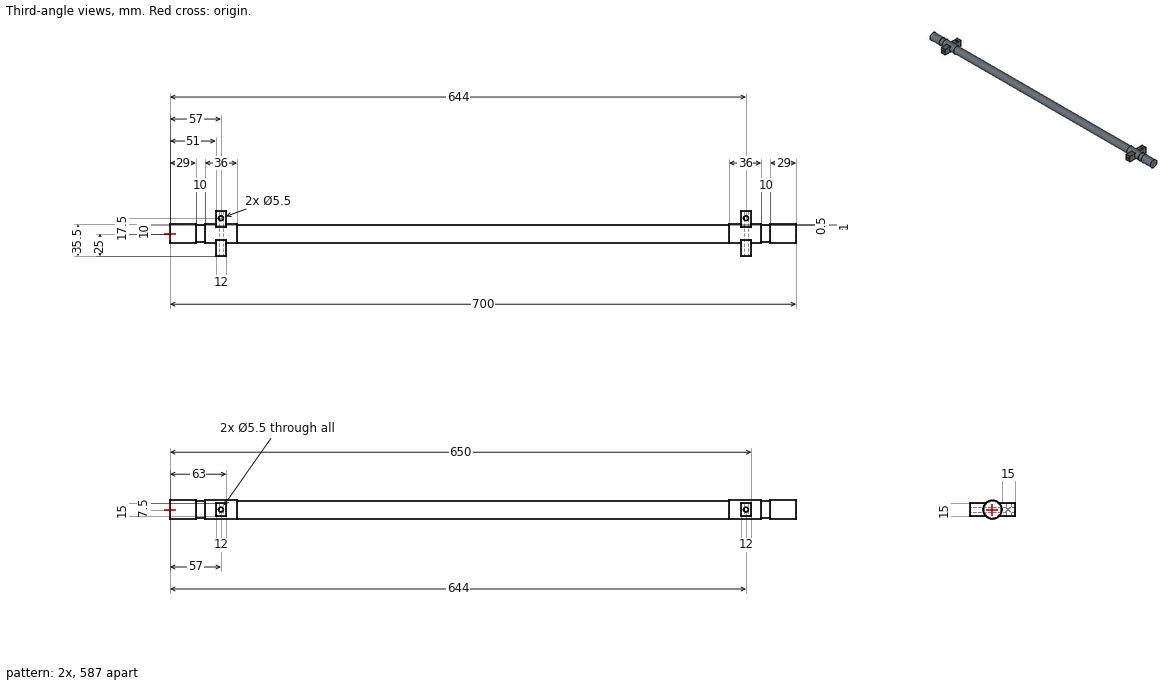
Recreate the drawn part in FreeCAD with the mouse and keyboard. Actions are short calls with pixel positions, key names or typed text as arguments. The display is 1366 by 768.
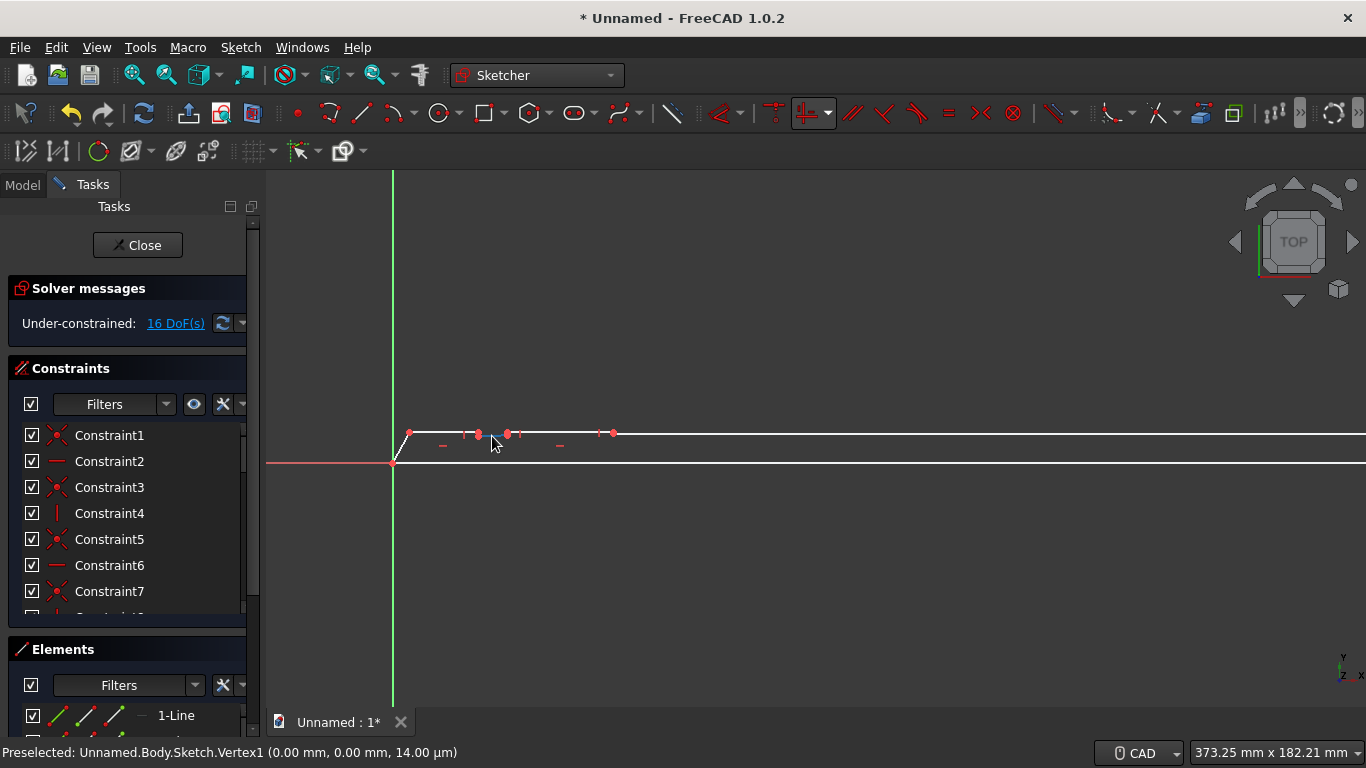
click(493, 436)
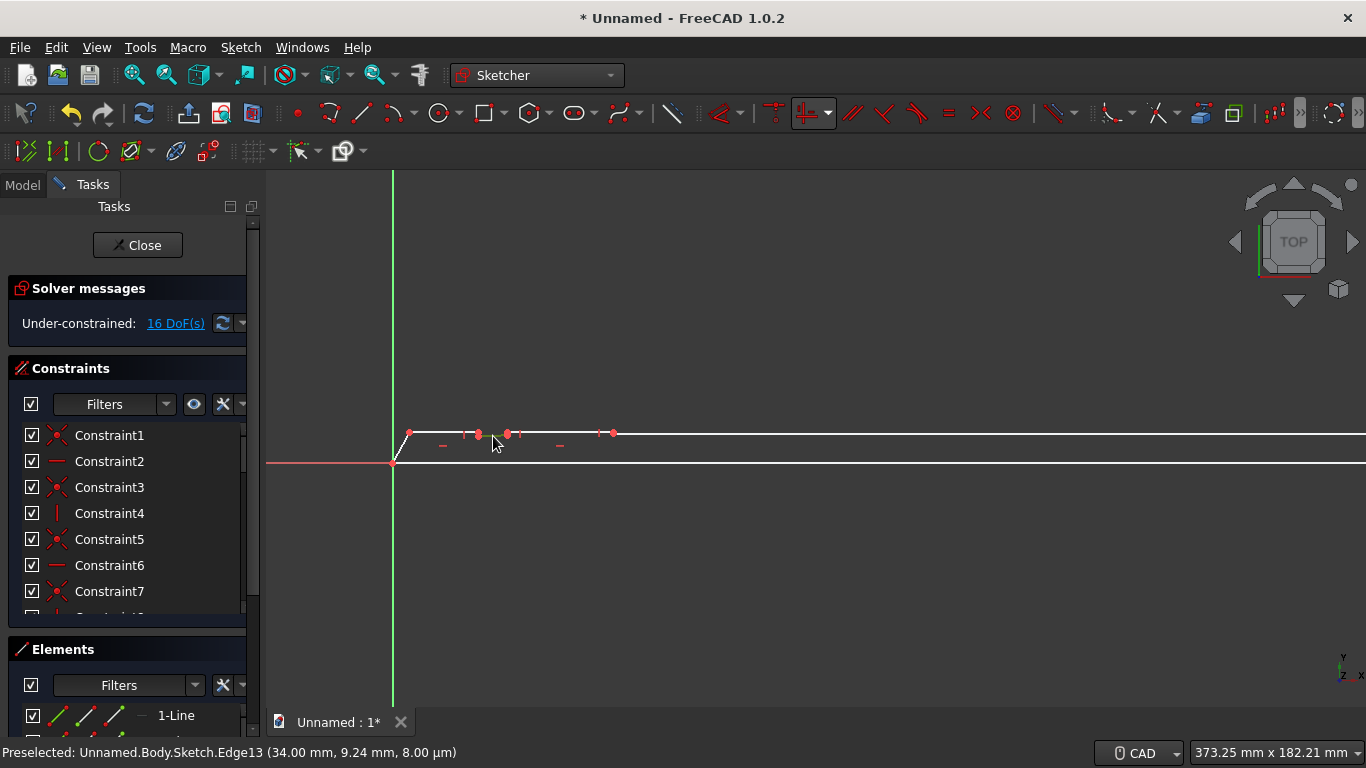
click(830, 114)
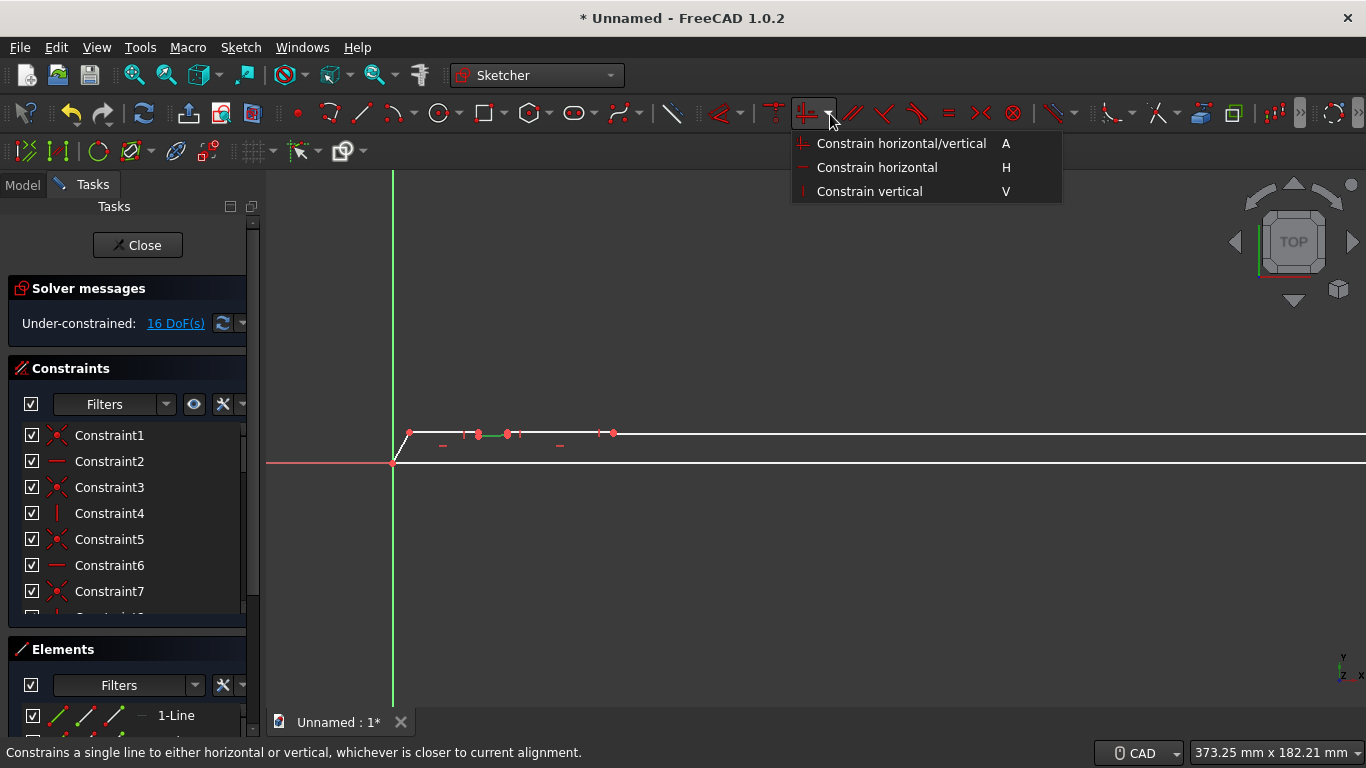
click(927, 167)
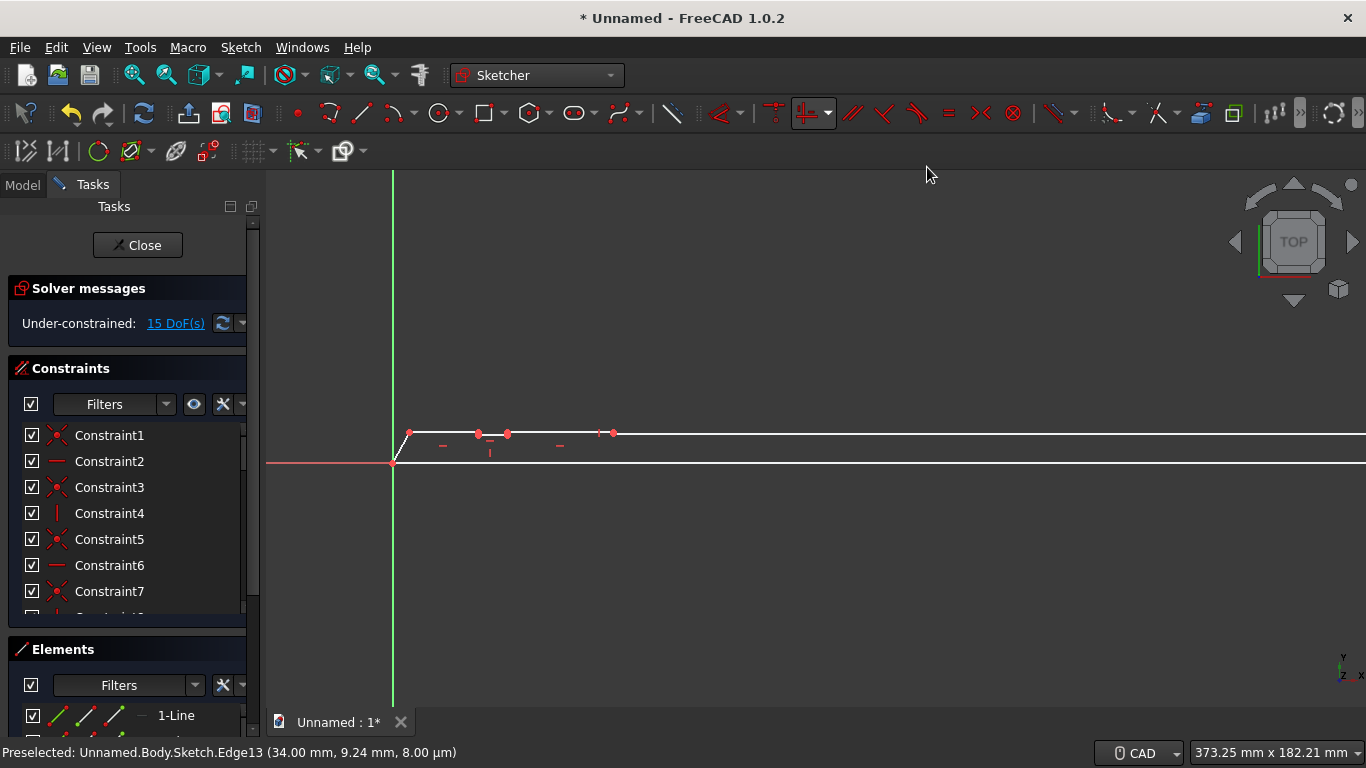
scroll(405, 442, up, 2)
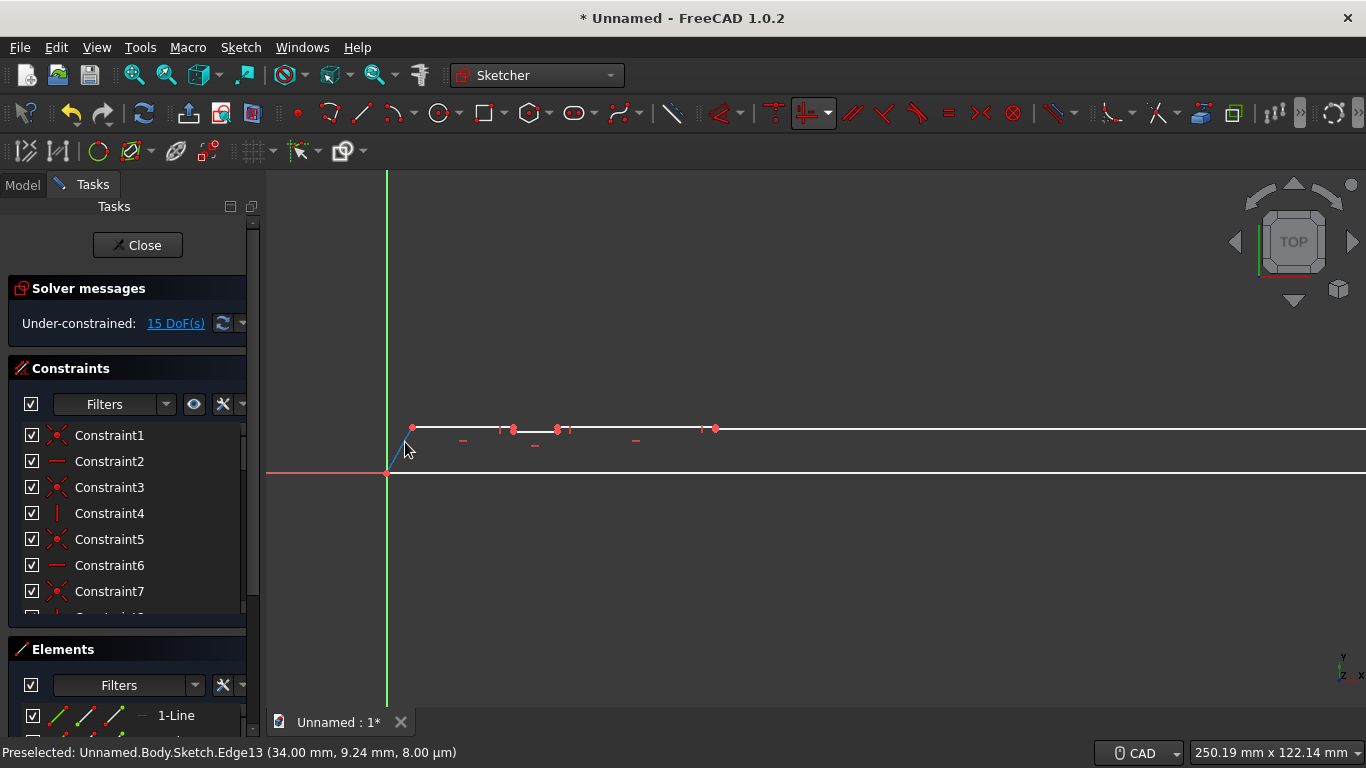
click(405, 441)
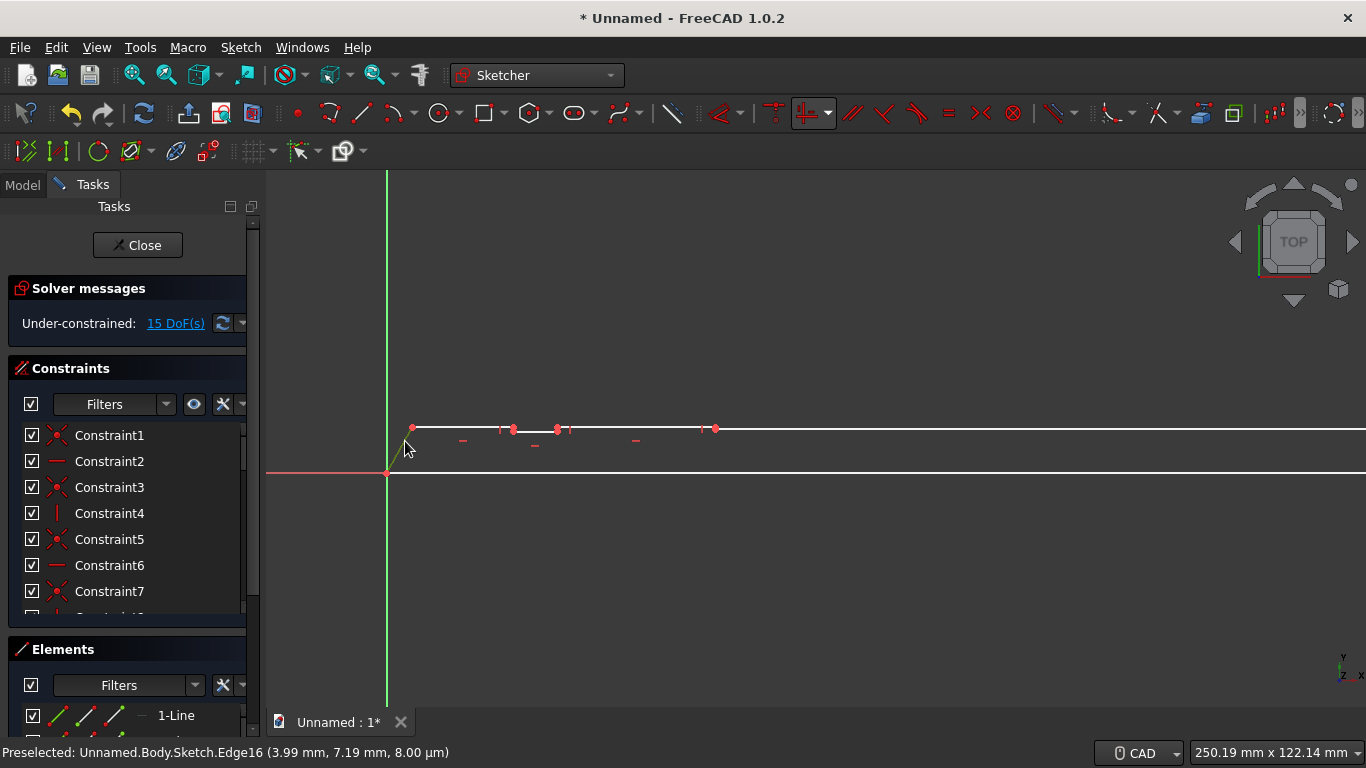
key(v)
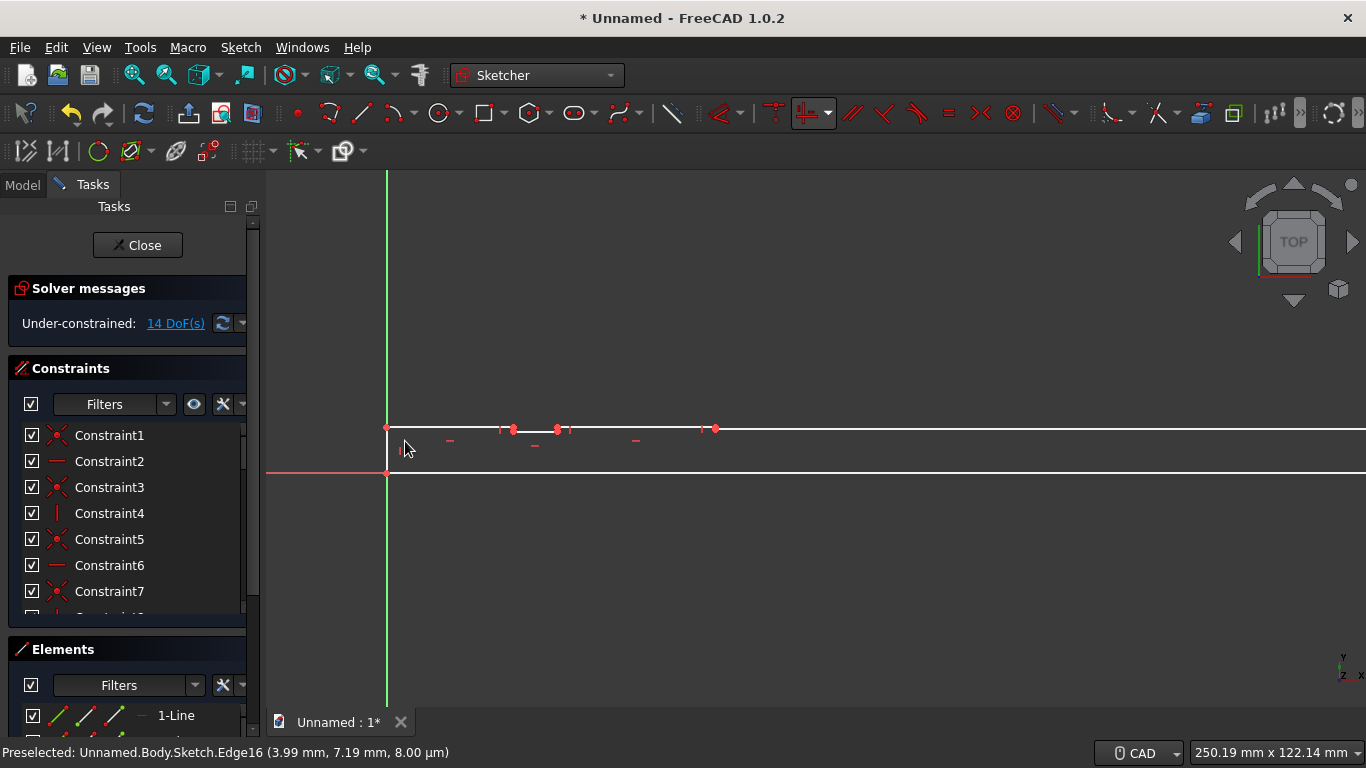
click(720, 114)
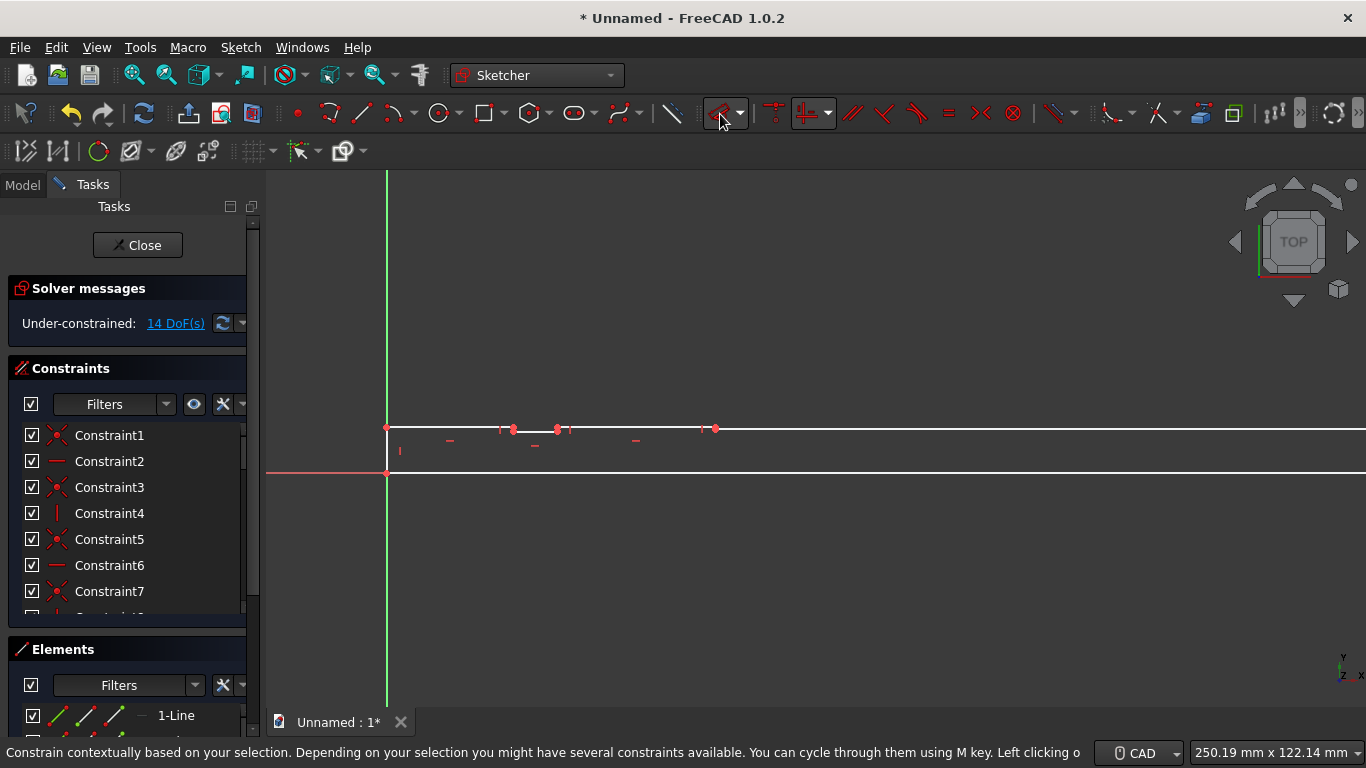
scroll(450, 436, down, 8)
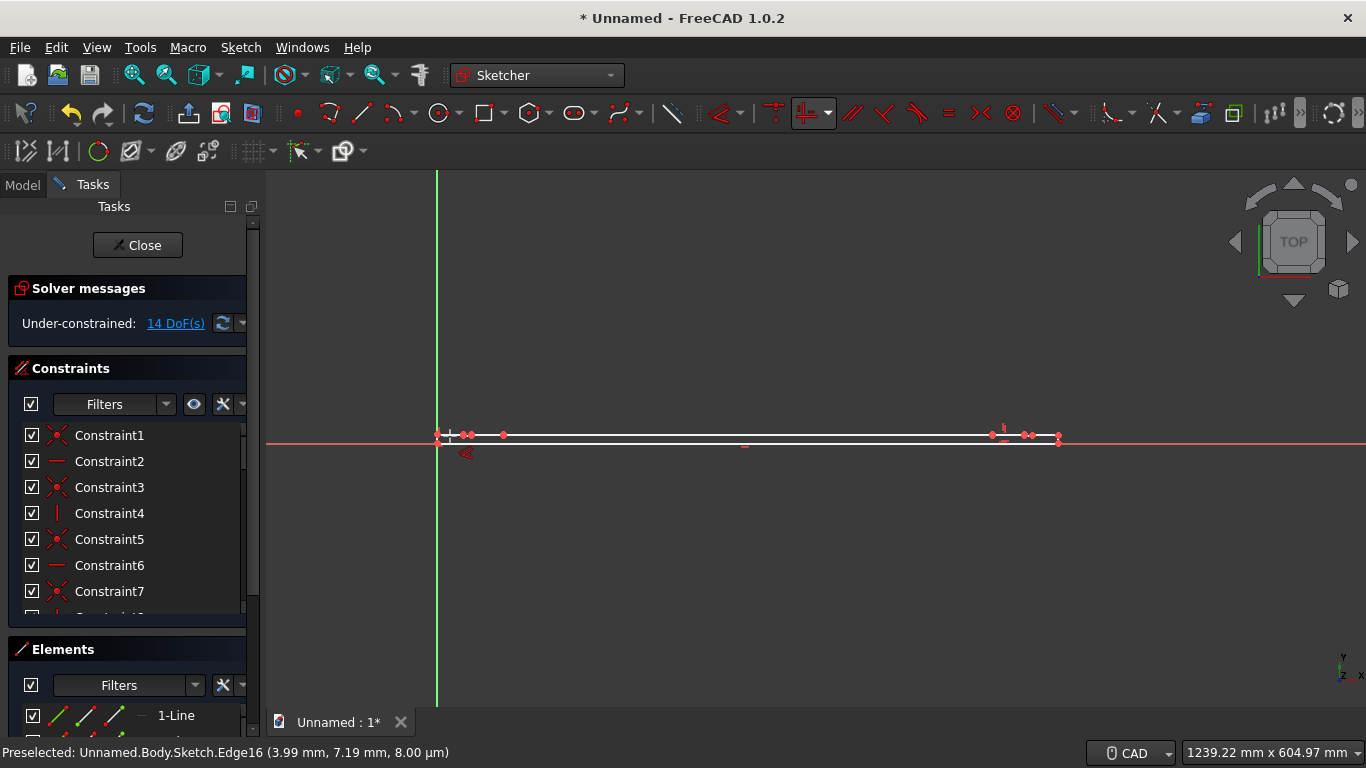
scroll(1033, 435, up, 20)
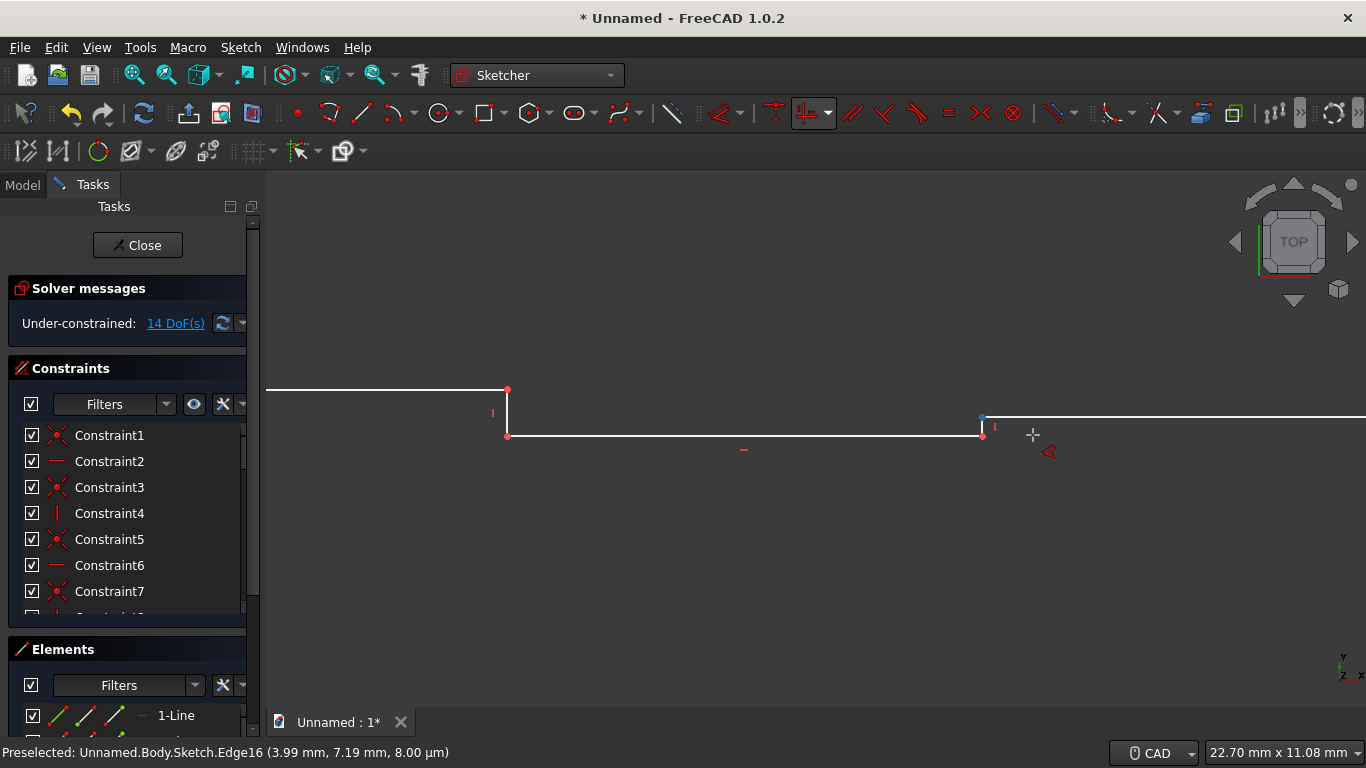
click(982, 427)
click(1016, 431)